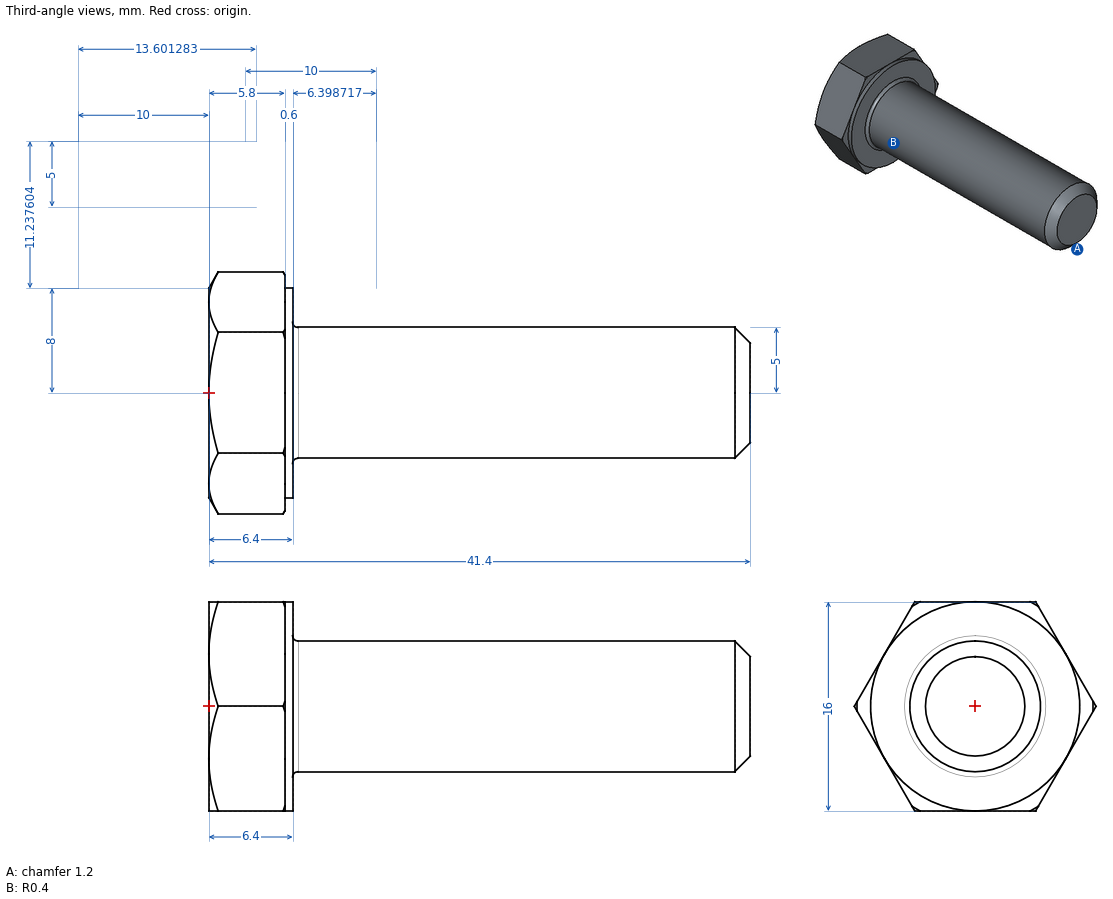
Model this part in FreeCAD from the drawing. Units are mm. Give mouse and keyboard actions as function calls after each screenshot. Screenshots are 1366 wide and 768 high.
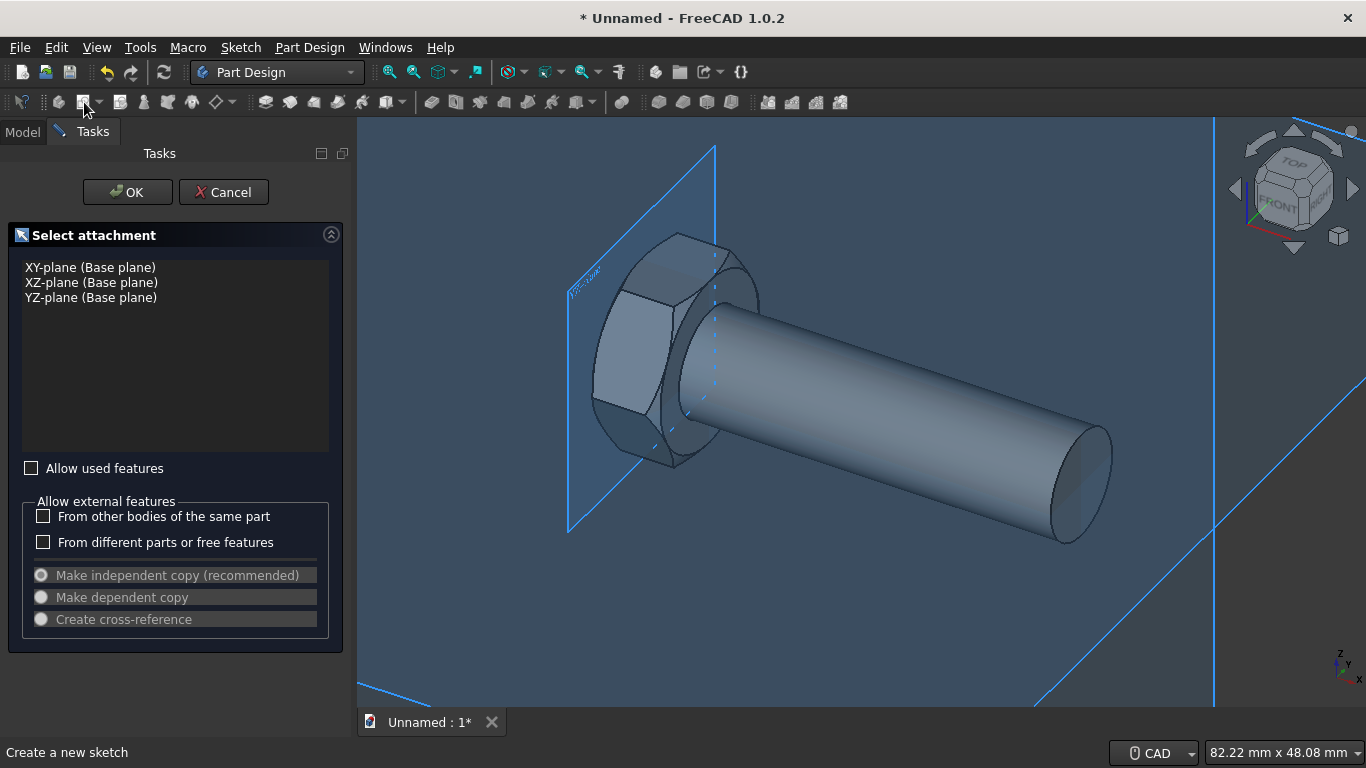
click(82, 268)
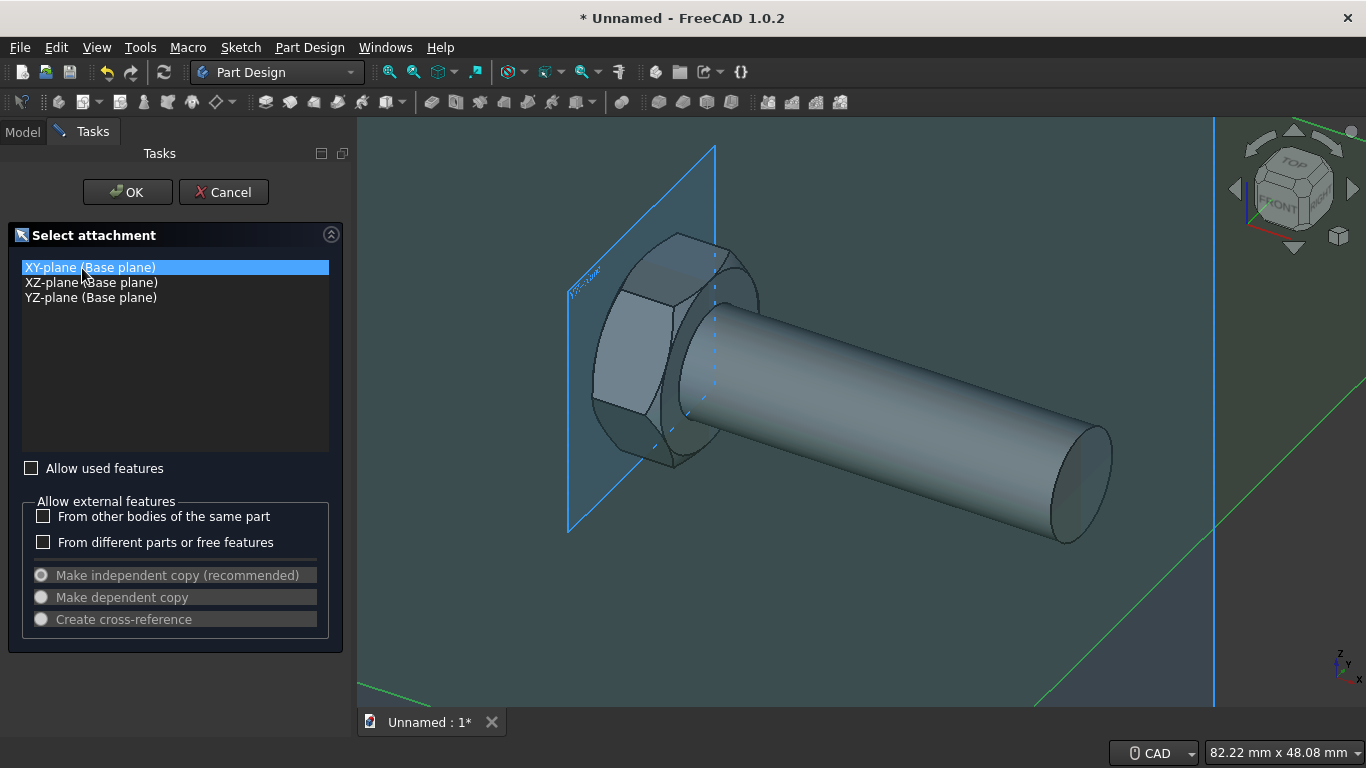
click(128, 192)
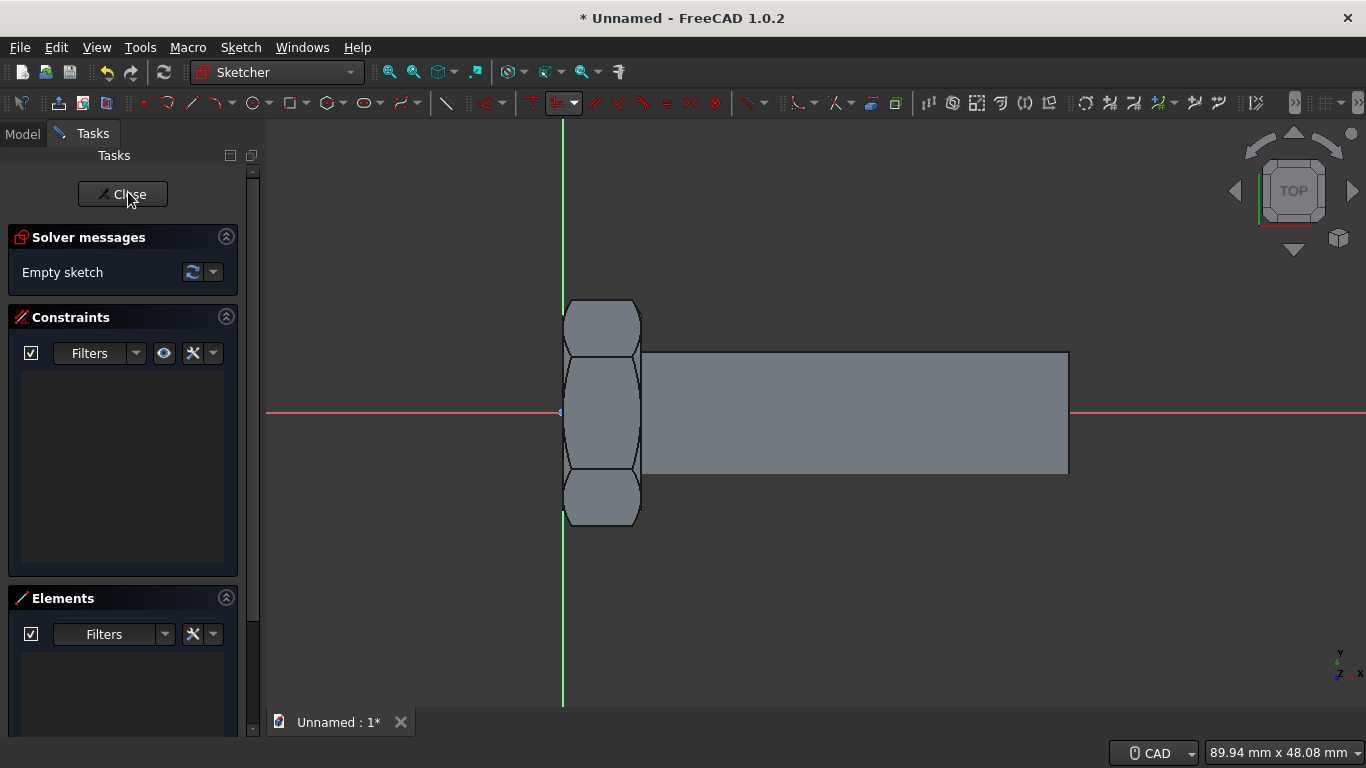
click(108, 104)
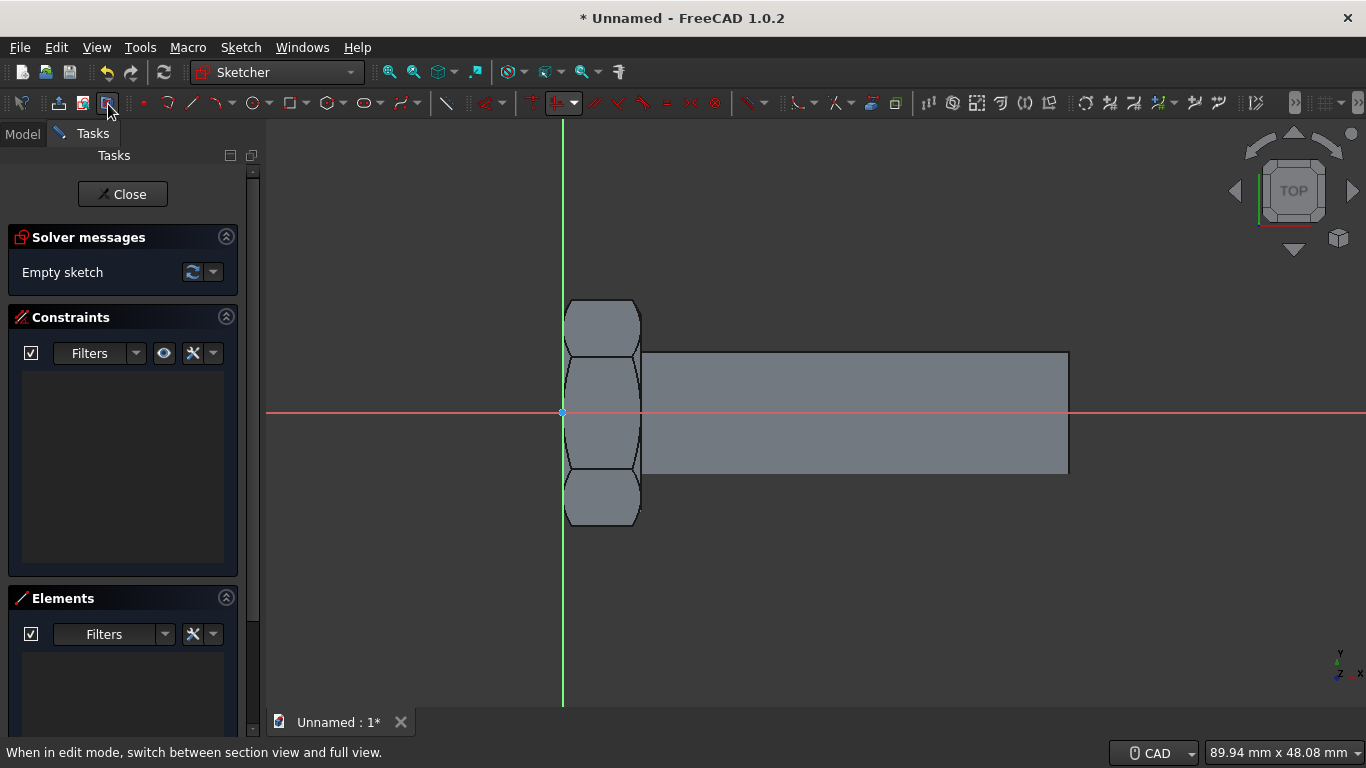
scroll(306, 147, up, 2)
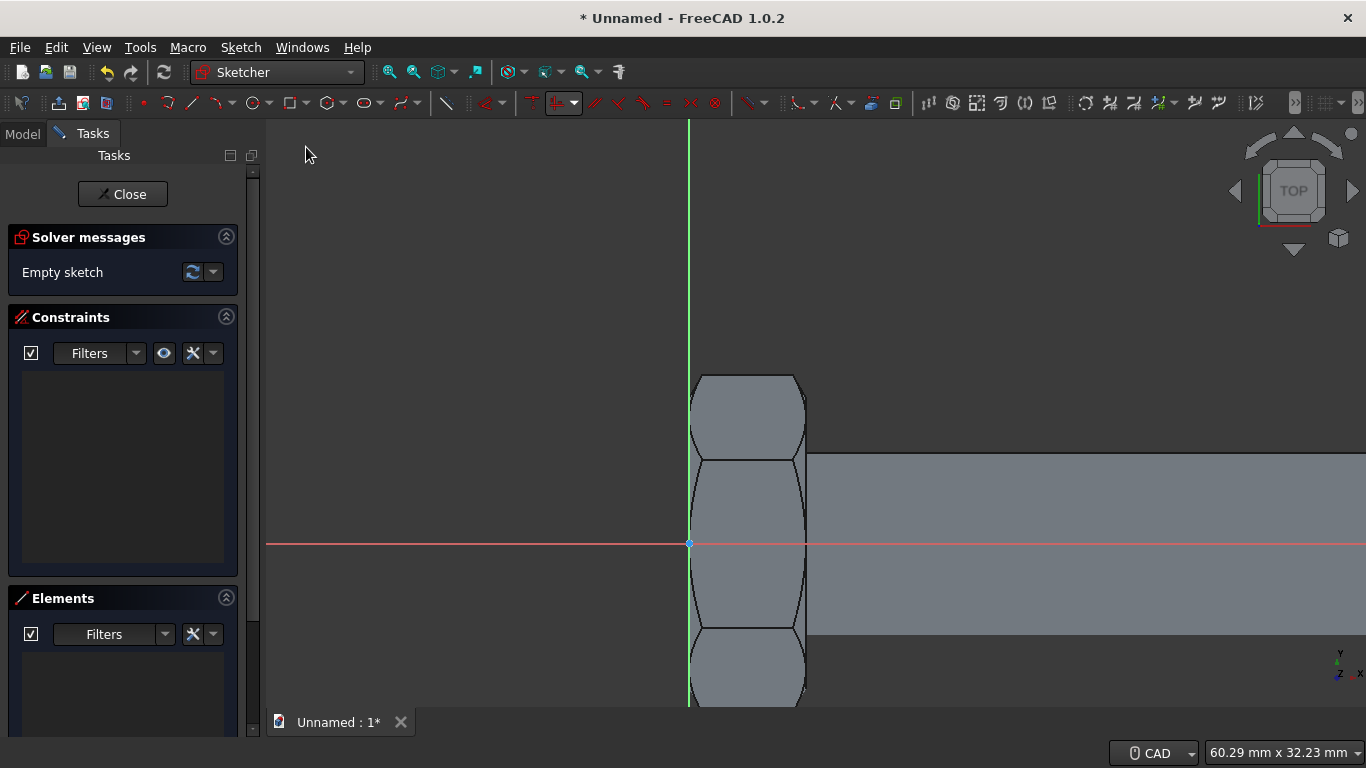
click(290, 104)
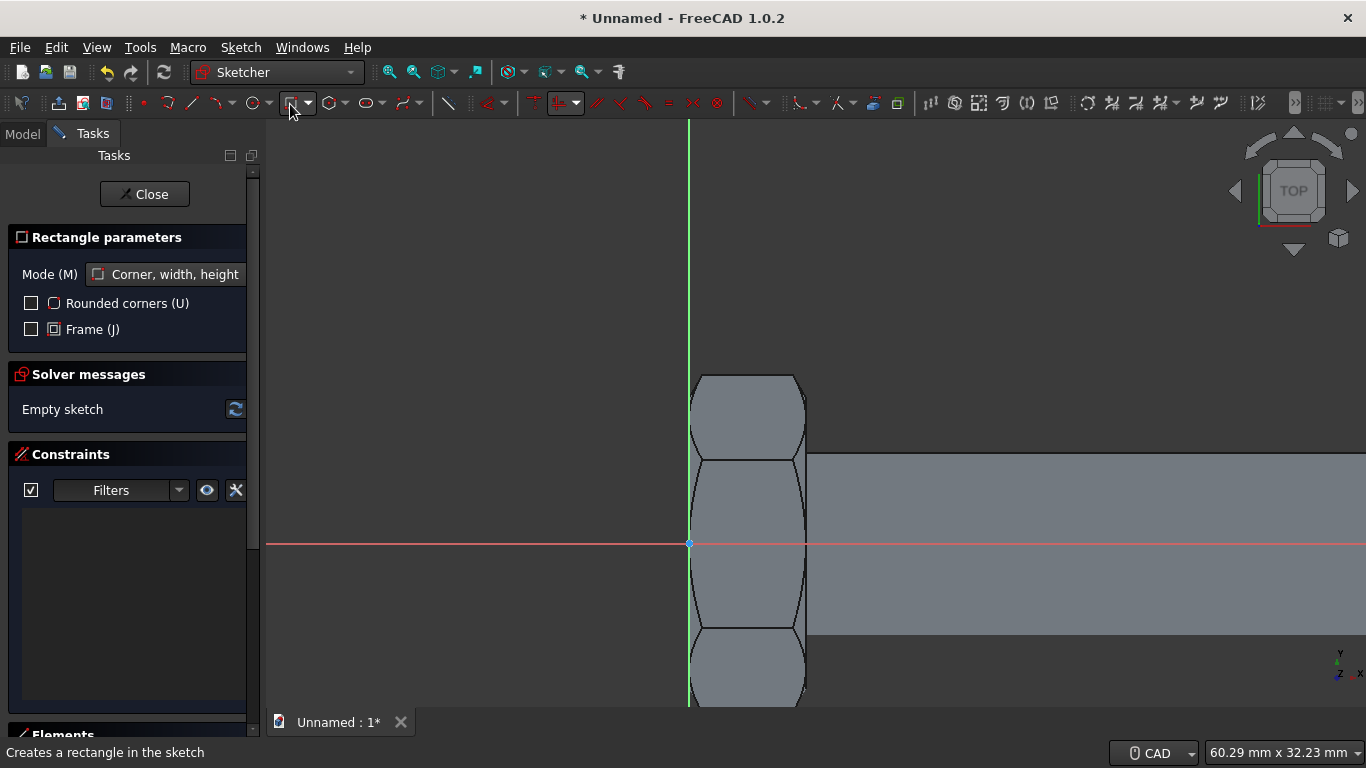
scroll(795, 193, up, 2)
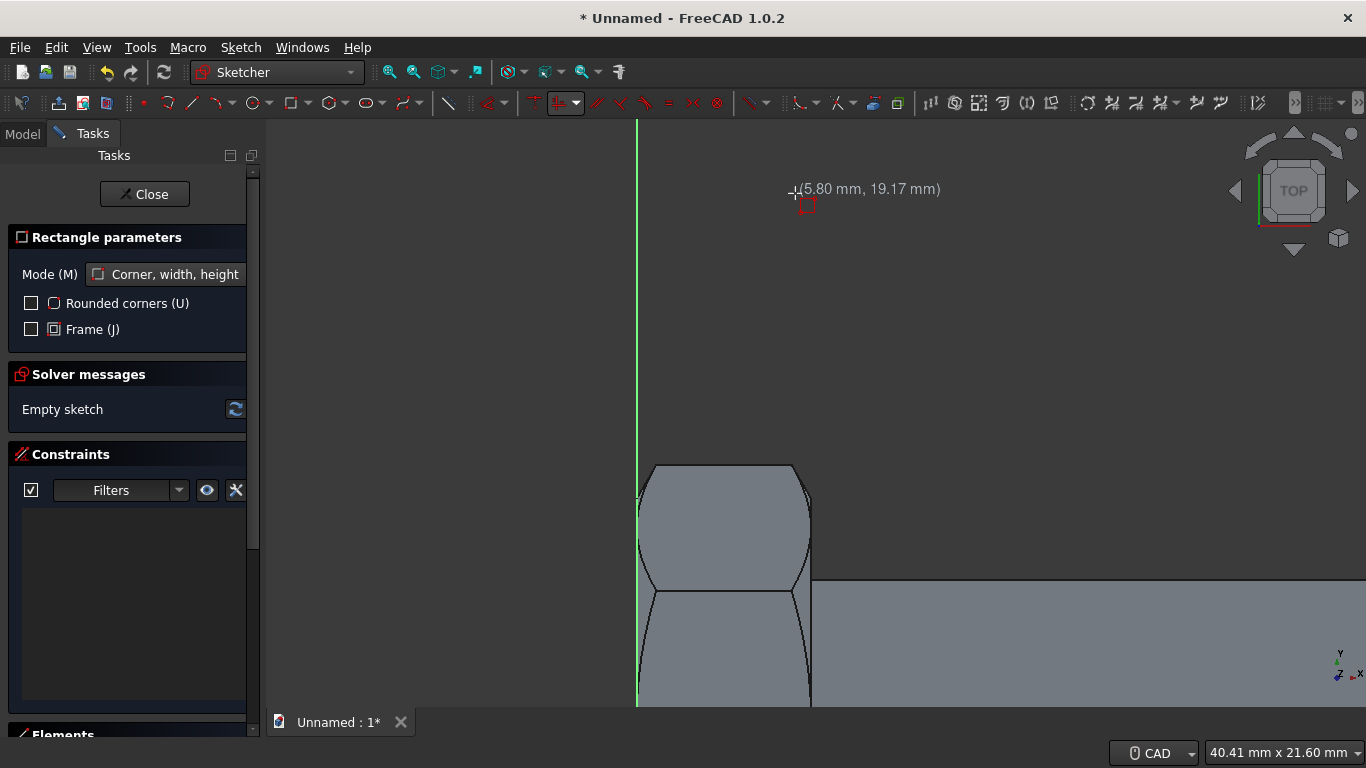
click(795, 193)
move(811, 499)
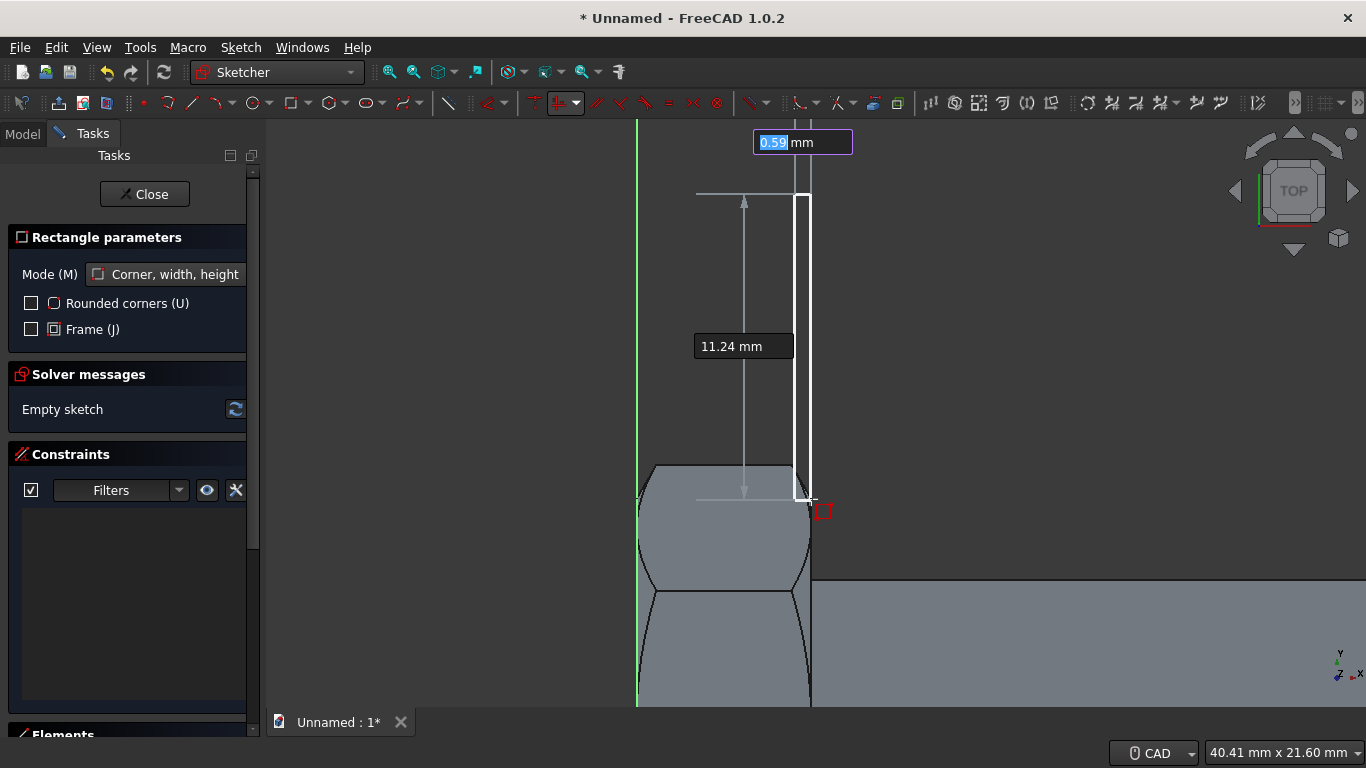
text(0.6)
key(Tab)
text(11.237604)
key(Return)
key(Escape)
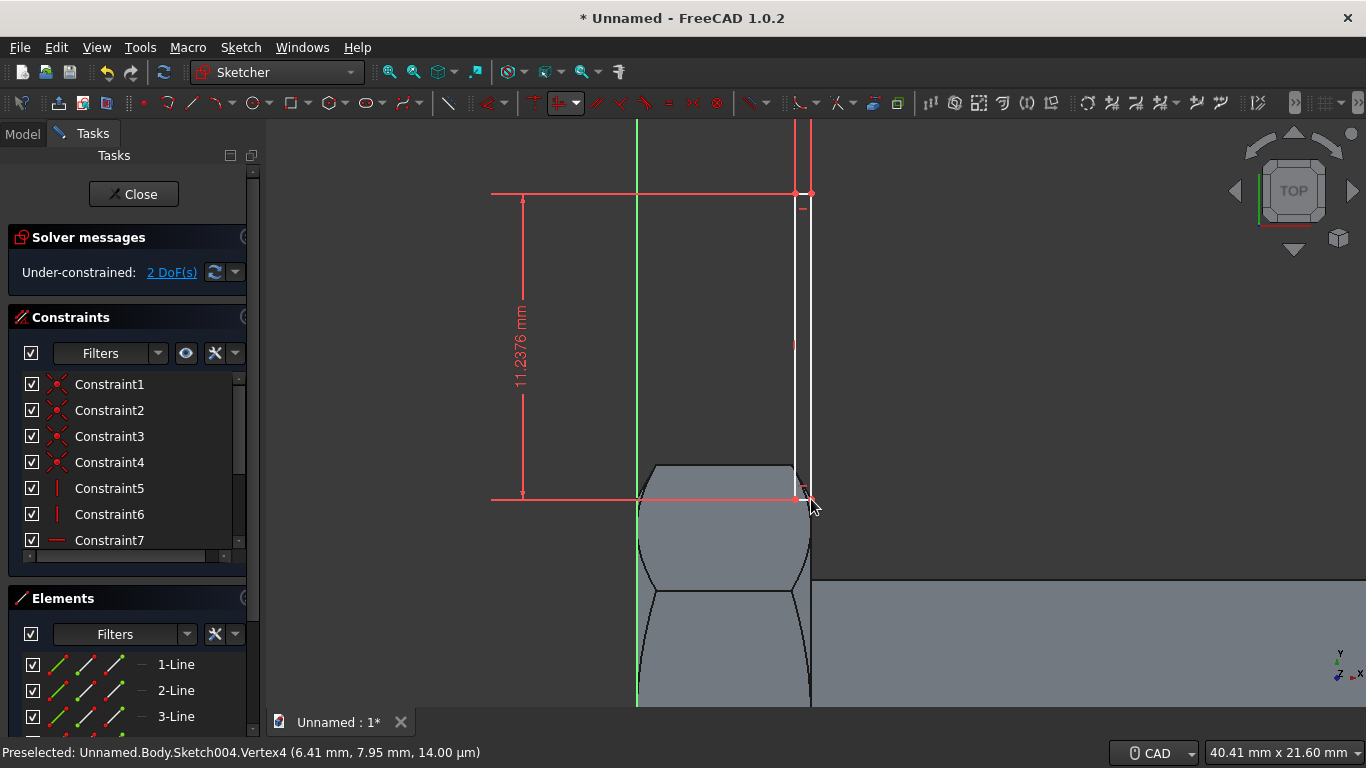
key(d)